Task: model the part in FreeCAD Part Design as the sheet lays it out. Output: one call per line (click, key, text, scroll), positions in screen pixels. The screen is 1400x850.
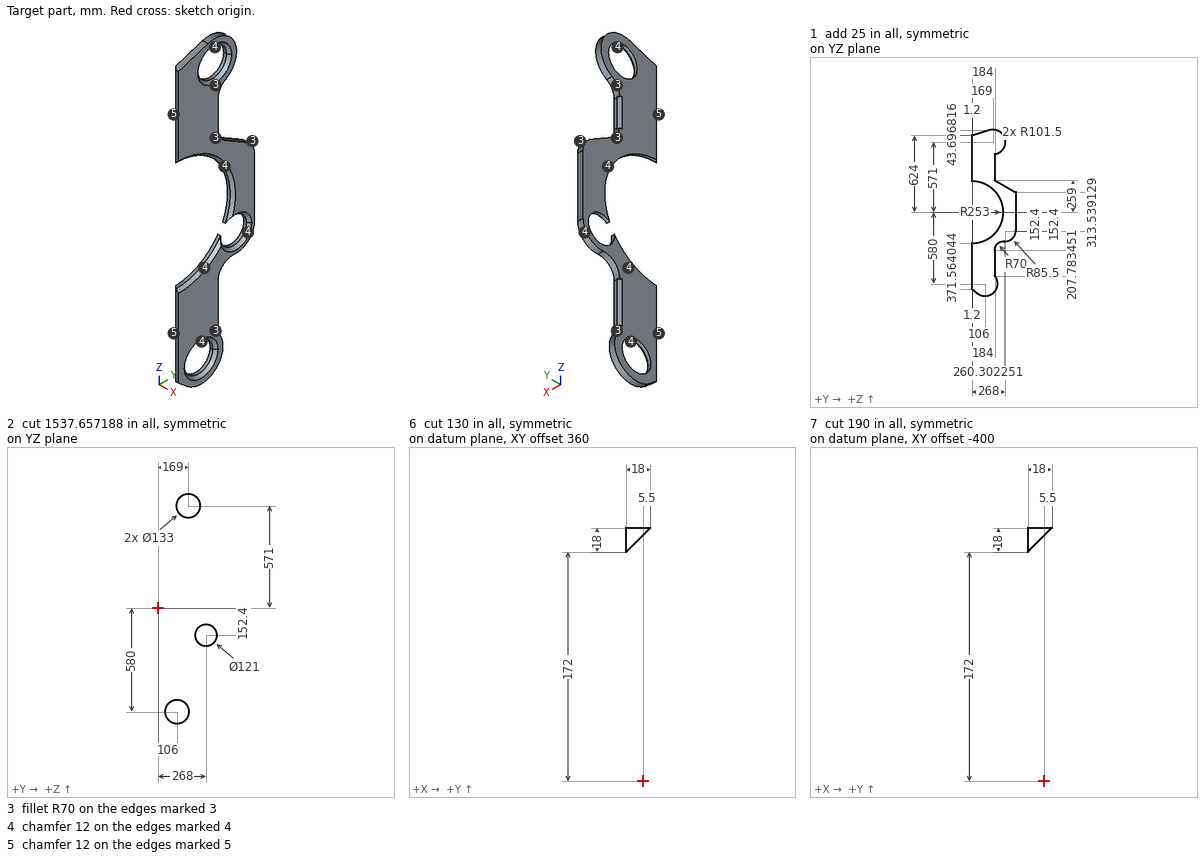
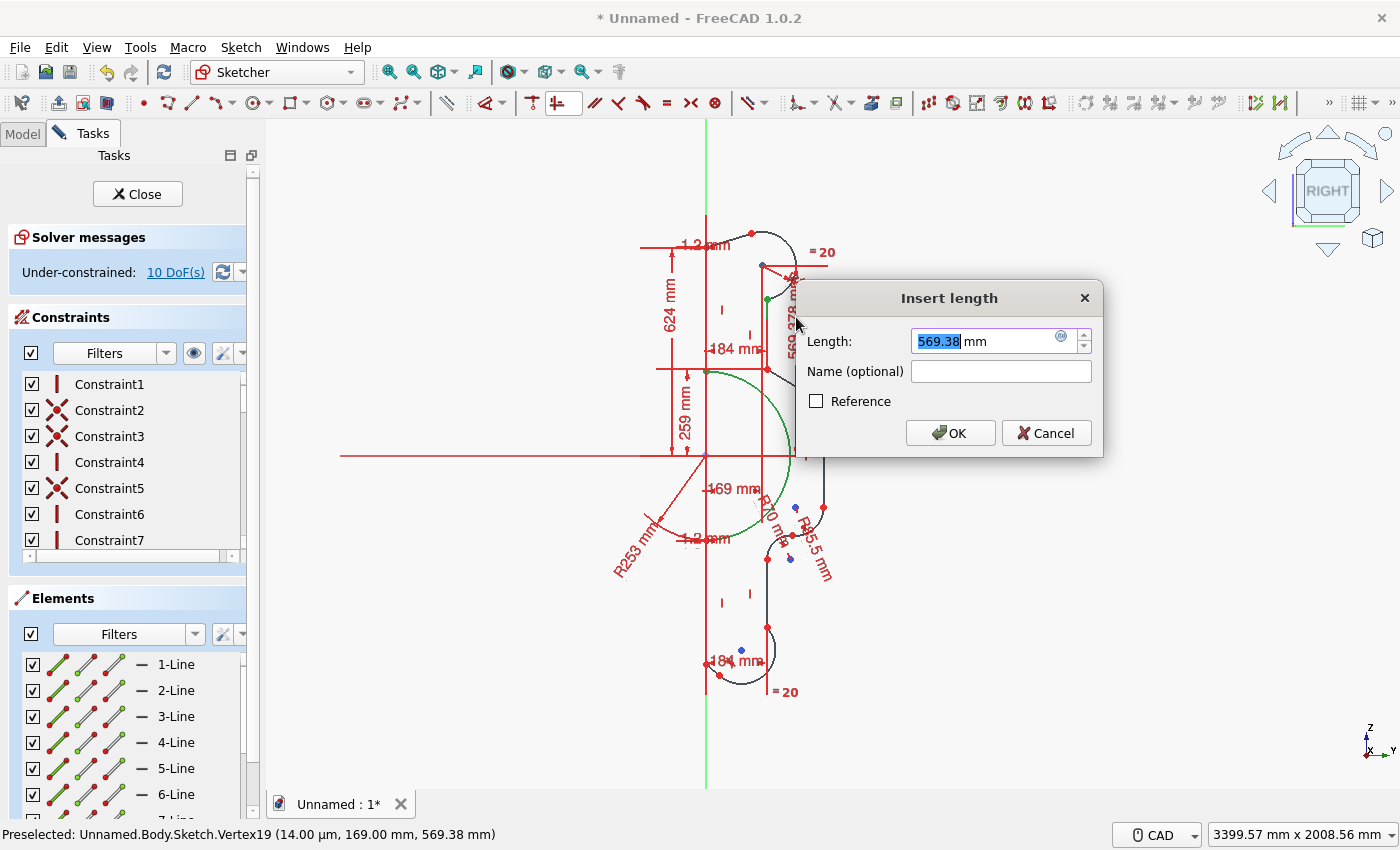
text(571)
key(Return)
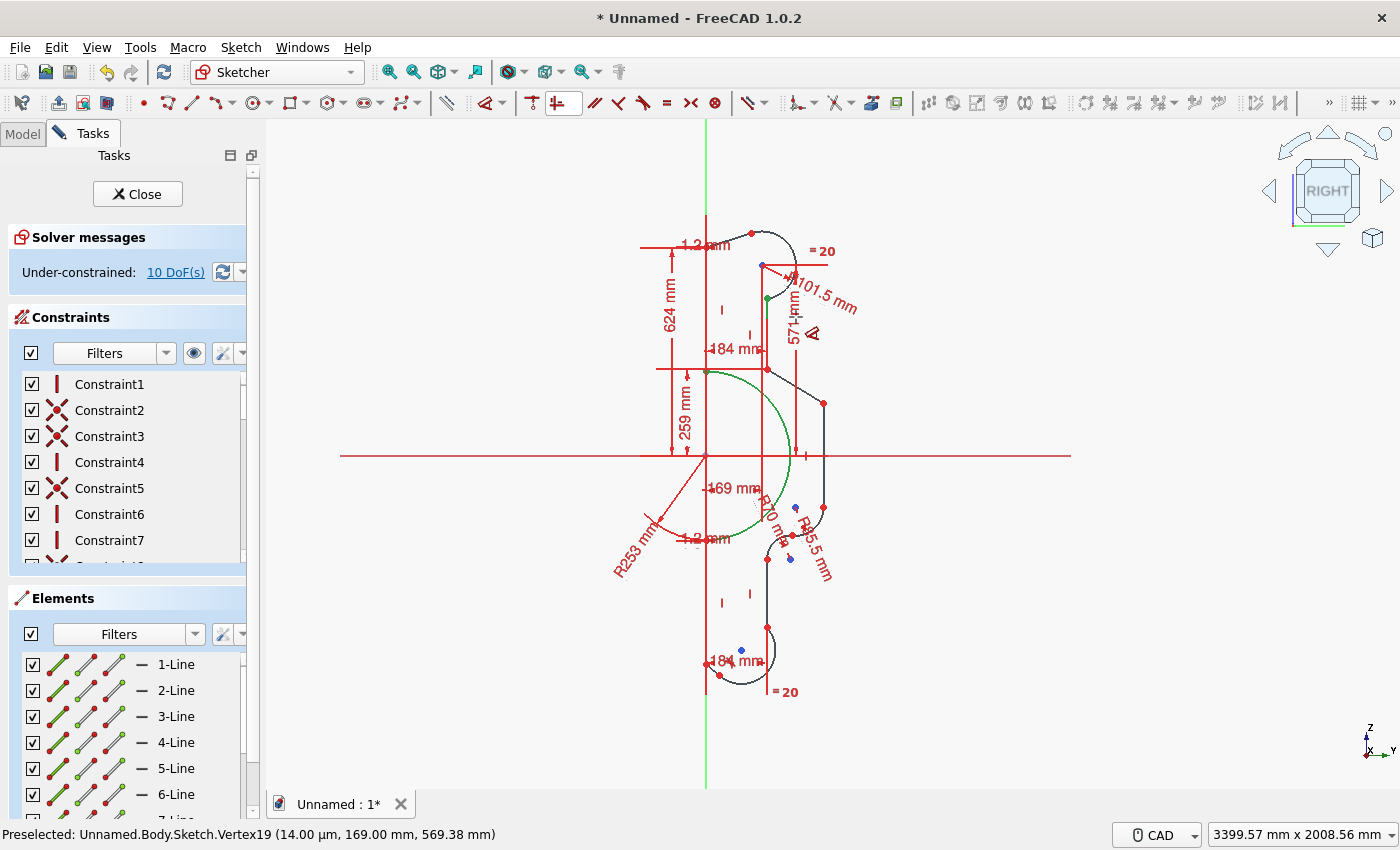
click(742, 650)
click(724, 708)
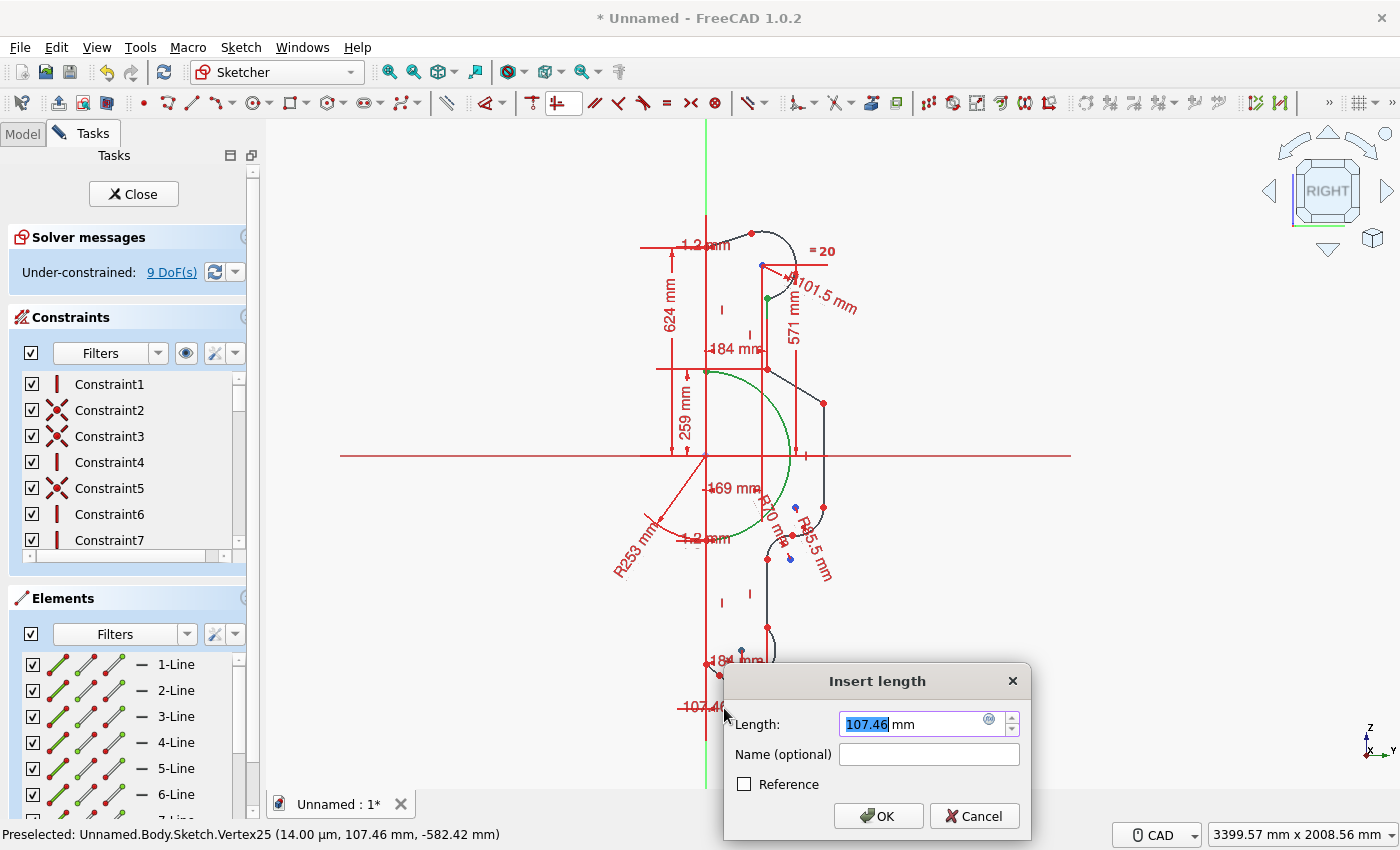
text(106)
key(Return)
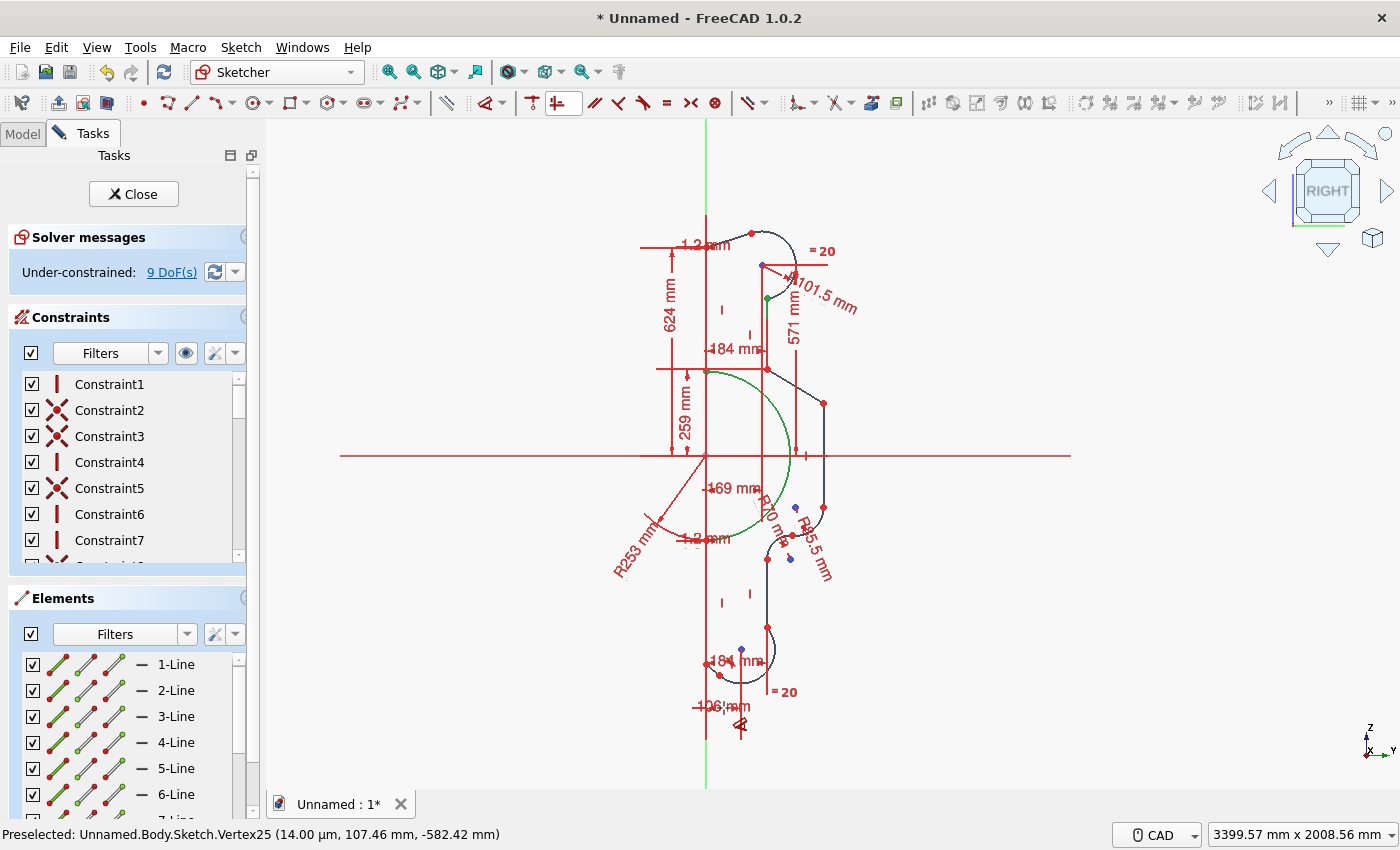
click(741, 650)
click(672, 597)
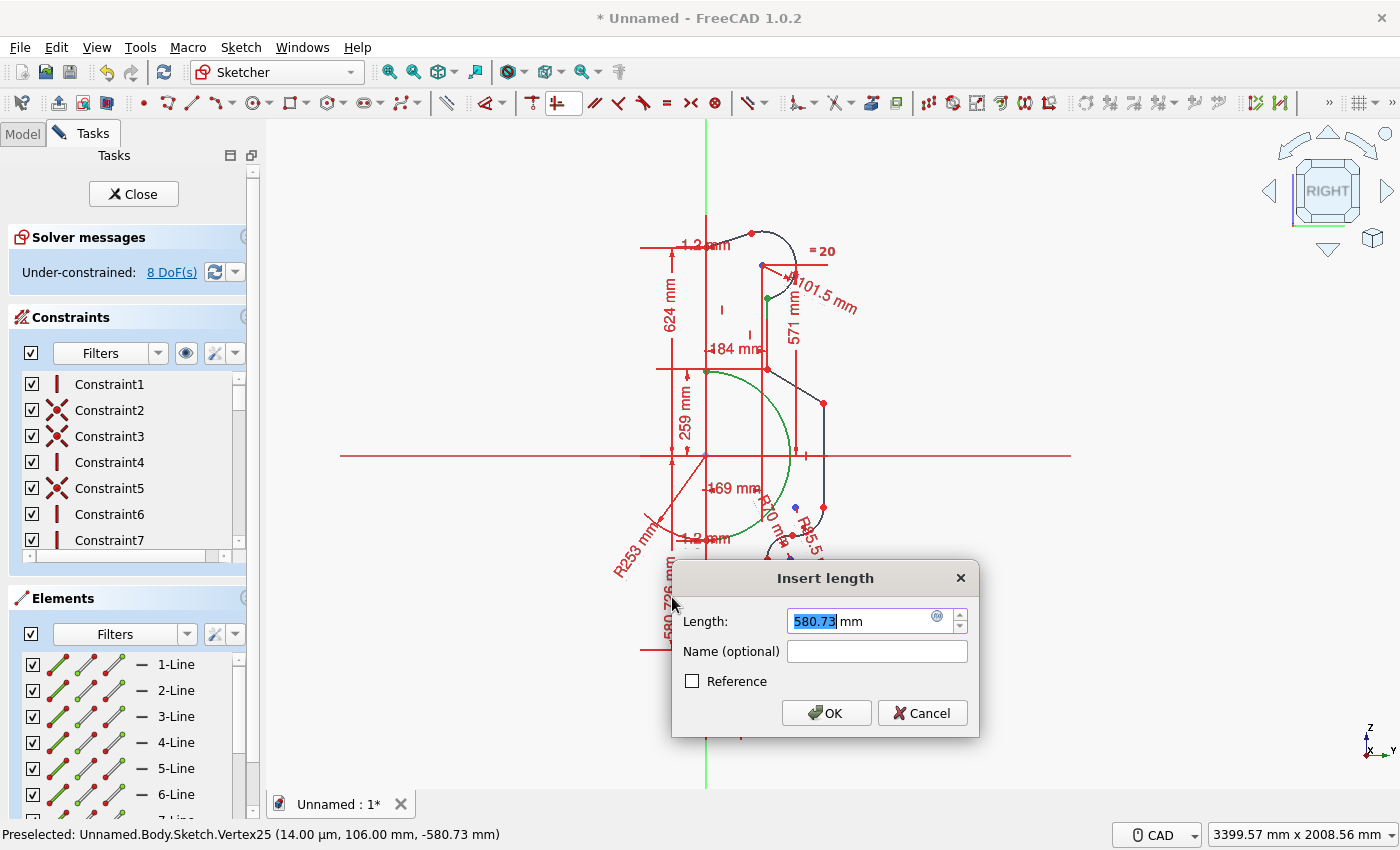
text(580)
key(Return)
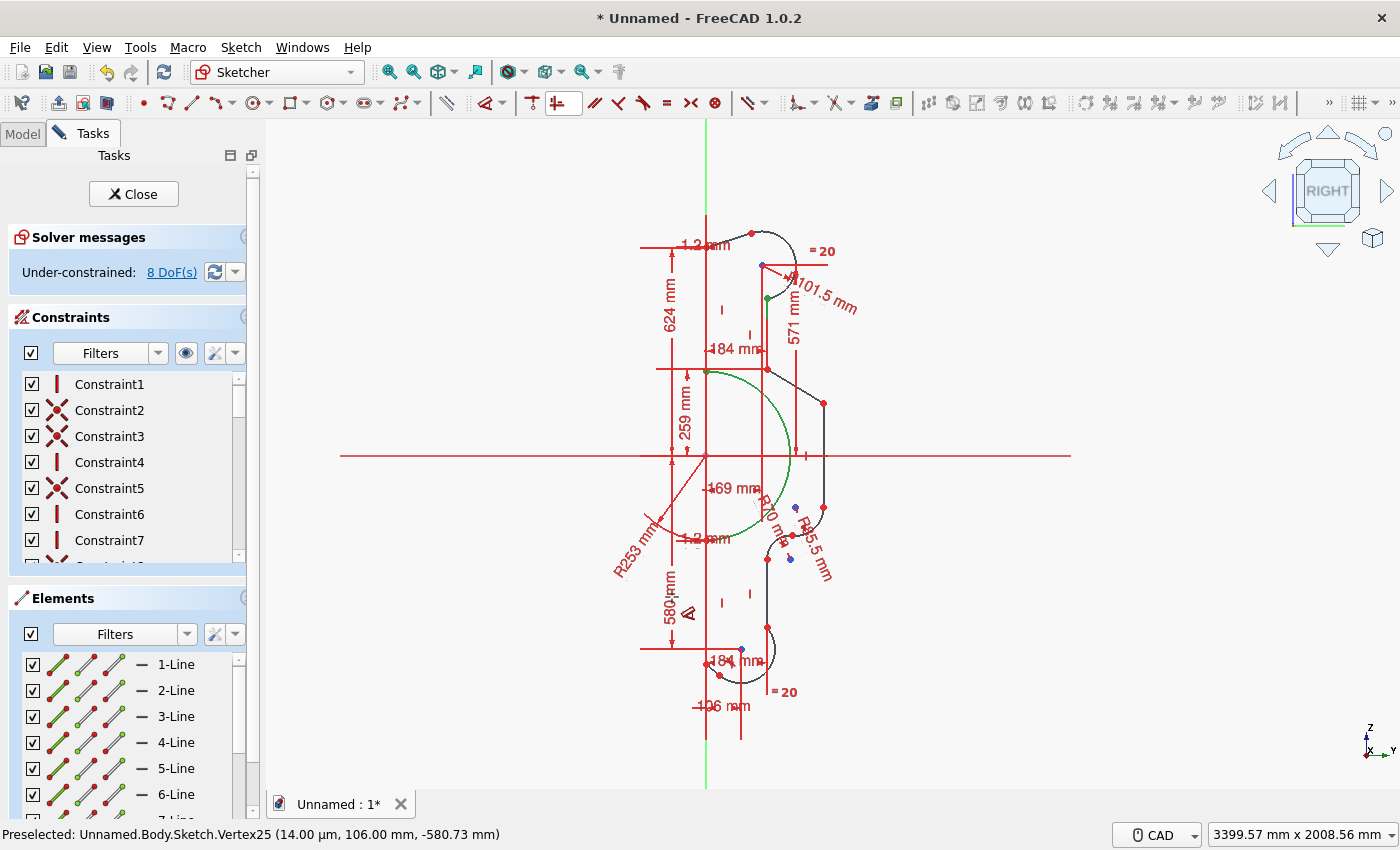
click(795, 507)
click(730, 565)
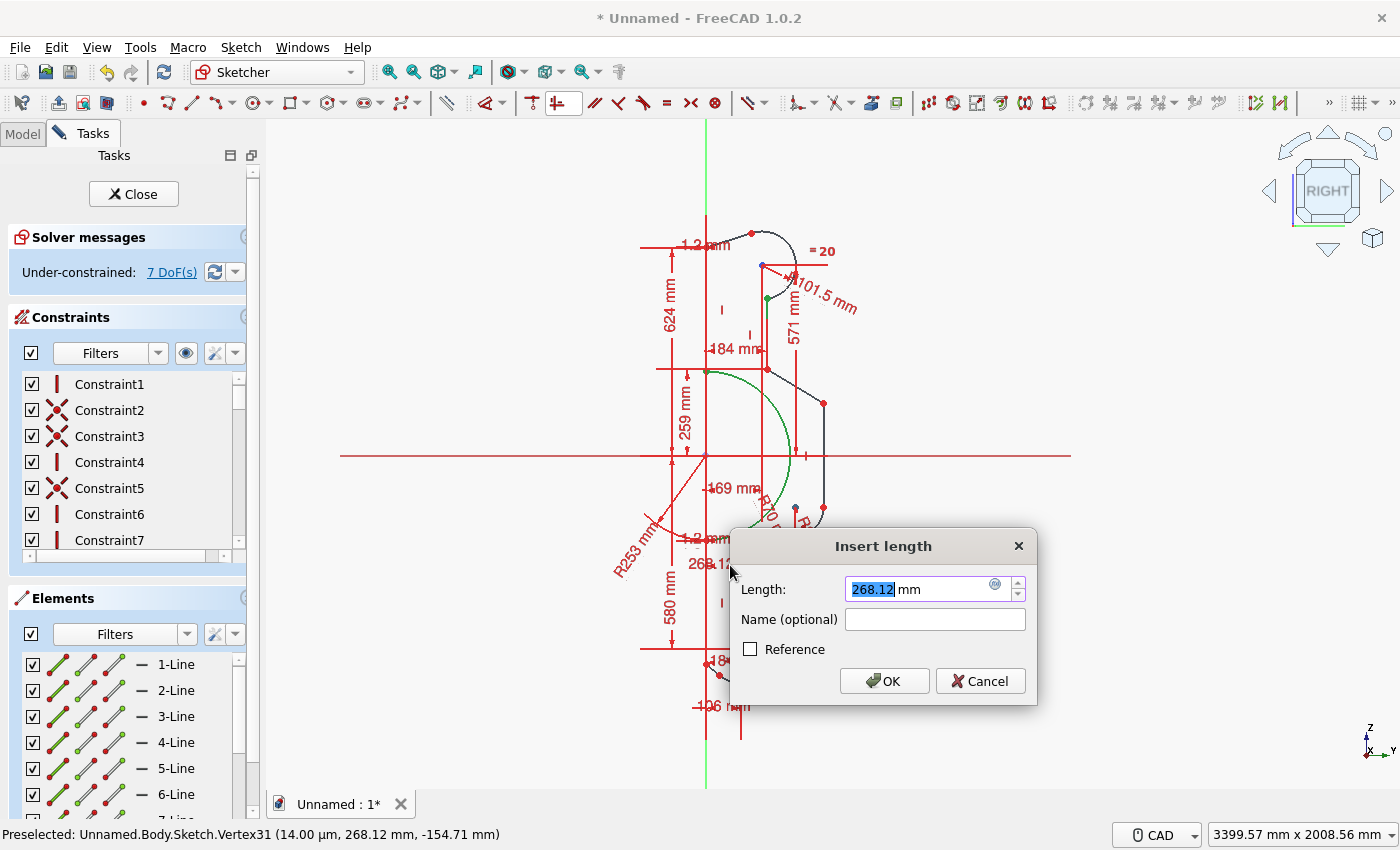
text(268)
key(Return)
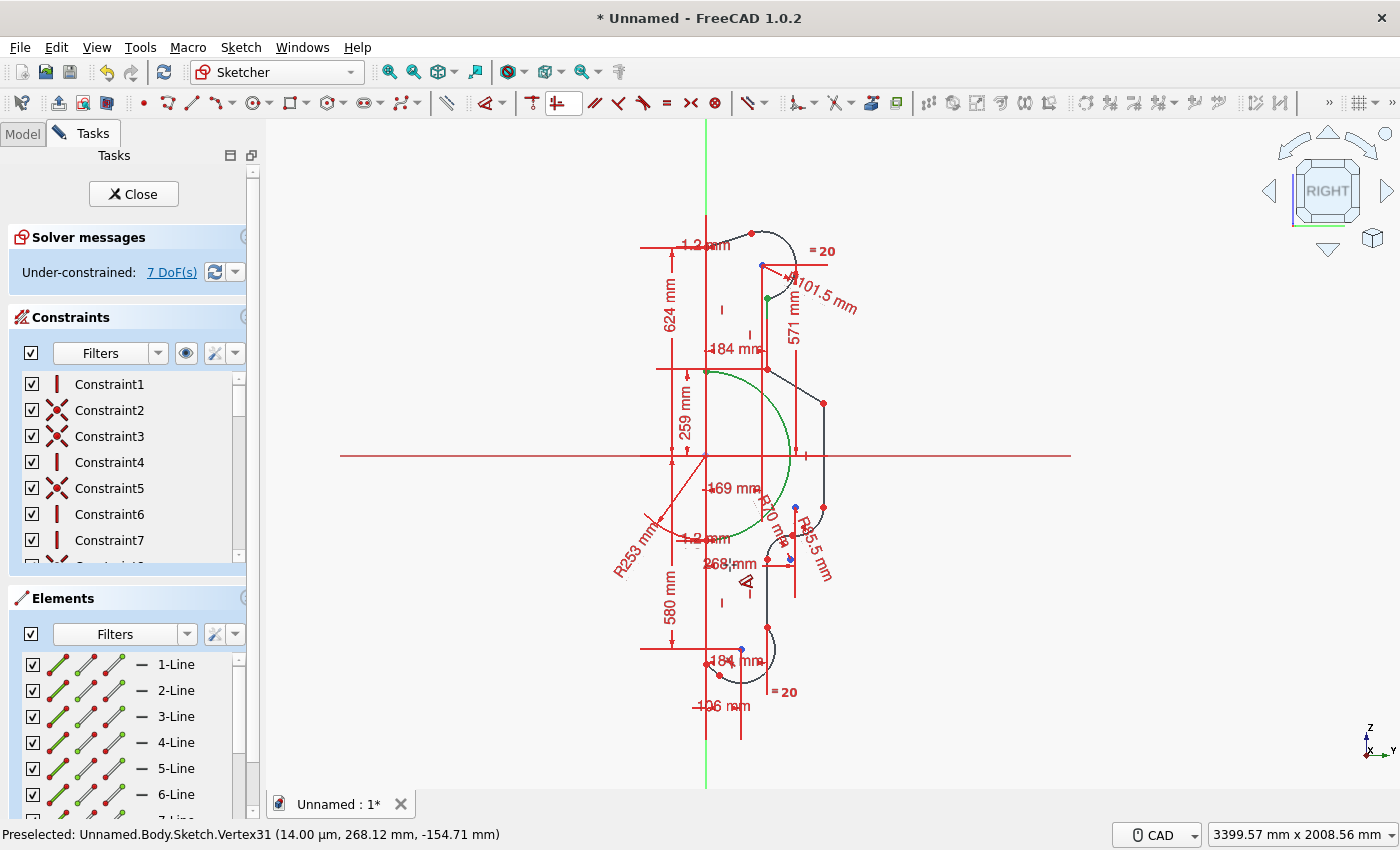
click(824, 507)
click(672, 470)